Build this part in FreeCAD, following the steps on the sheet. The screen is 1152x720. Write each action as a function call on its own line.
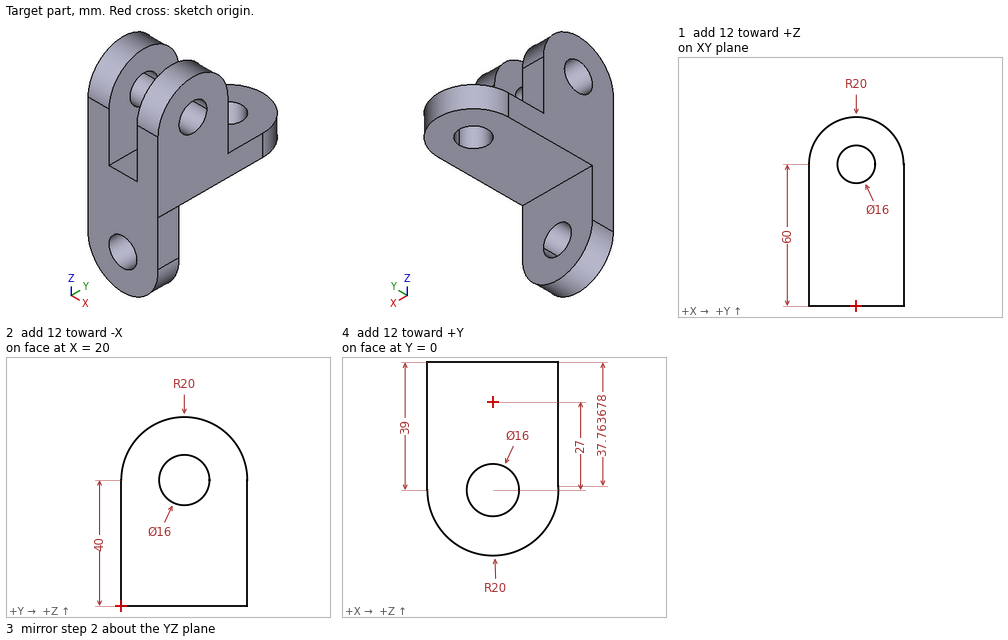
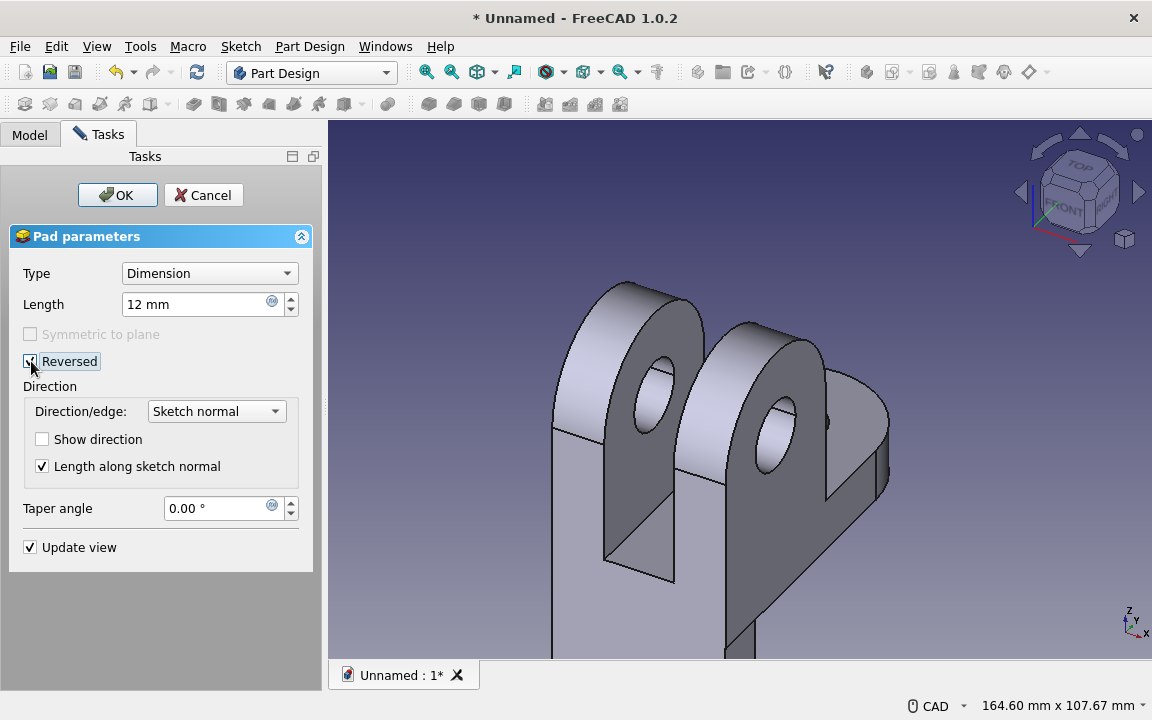
click(118, 195)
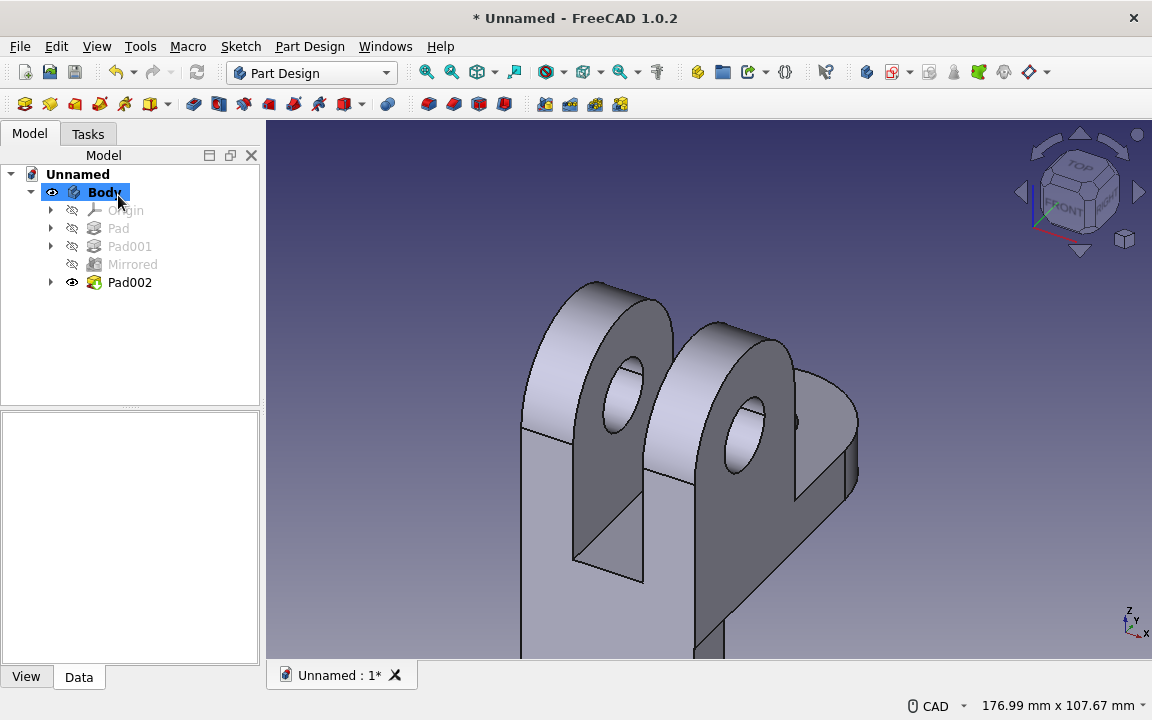
key(0)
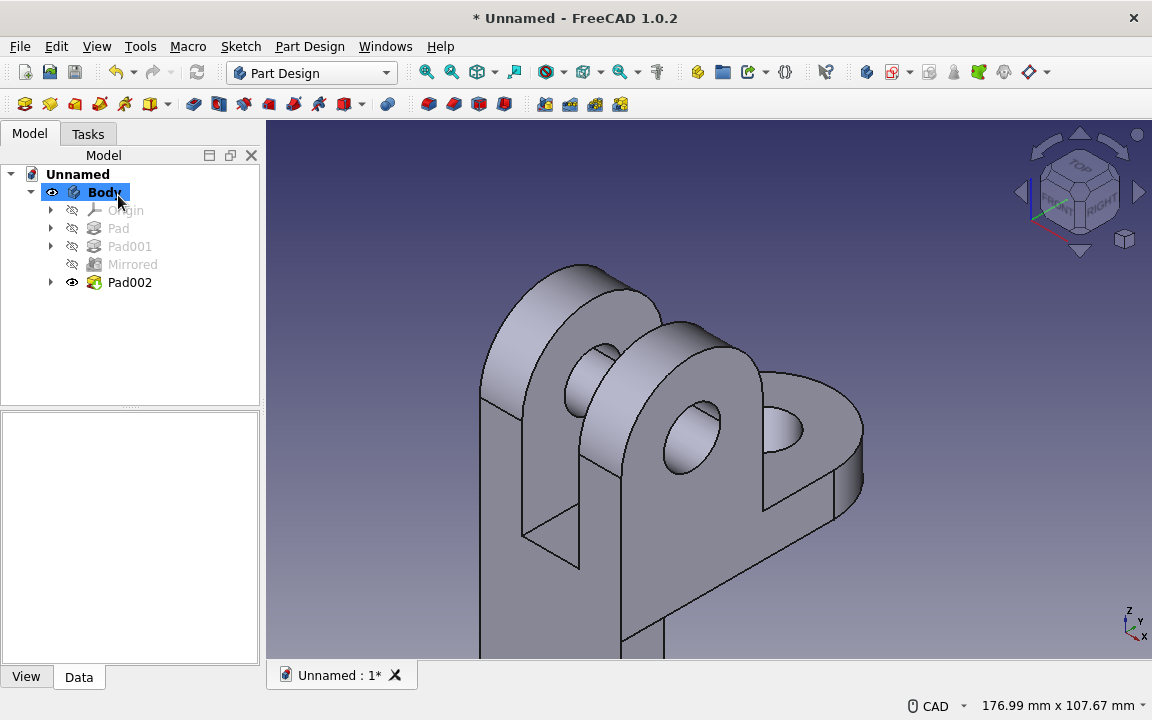
click(427, 72)